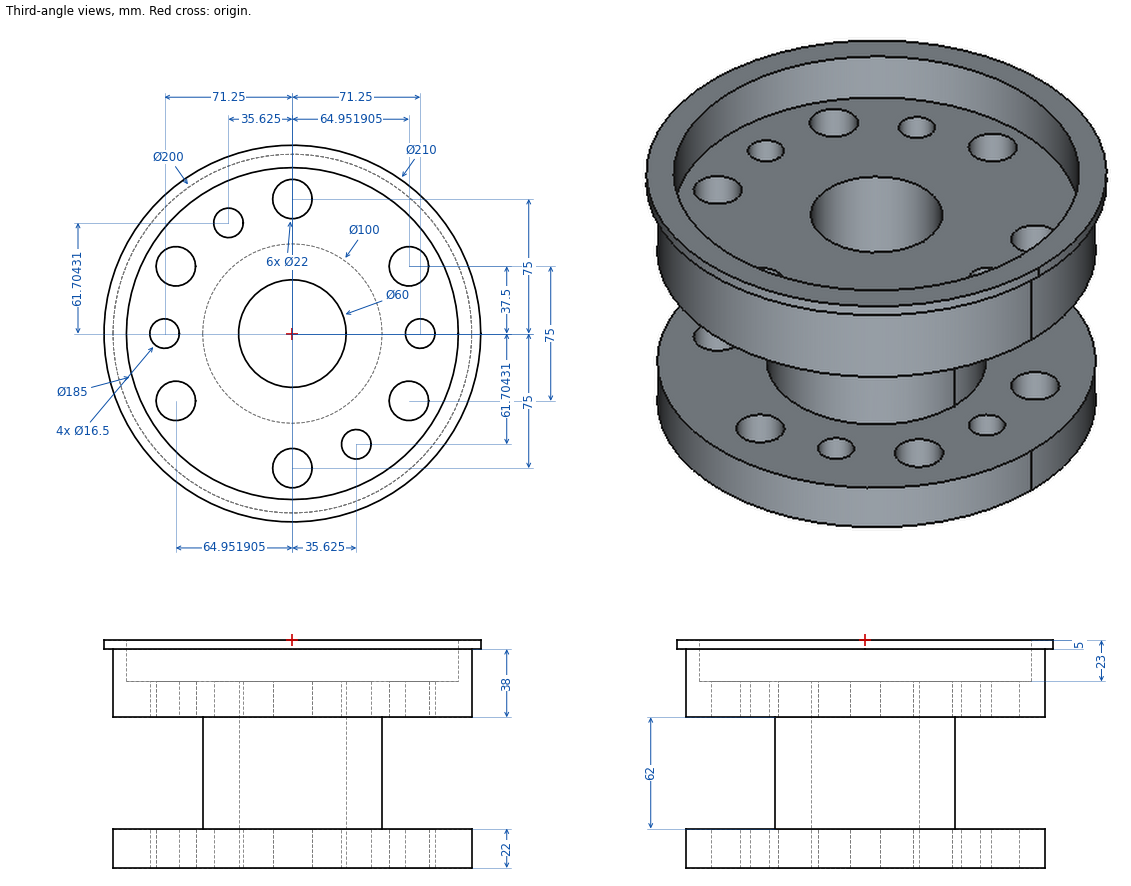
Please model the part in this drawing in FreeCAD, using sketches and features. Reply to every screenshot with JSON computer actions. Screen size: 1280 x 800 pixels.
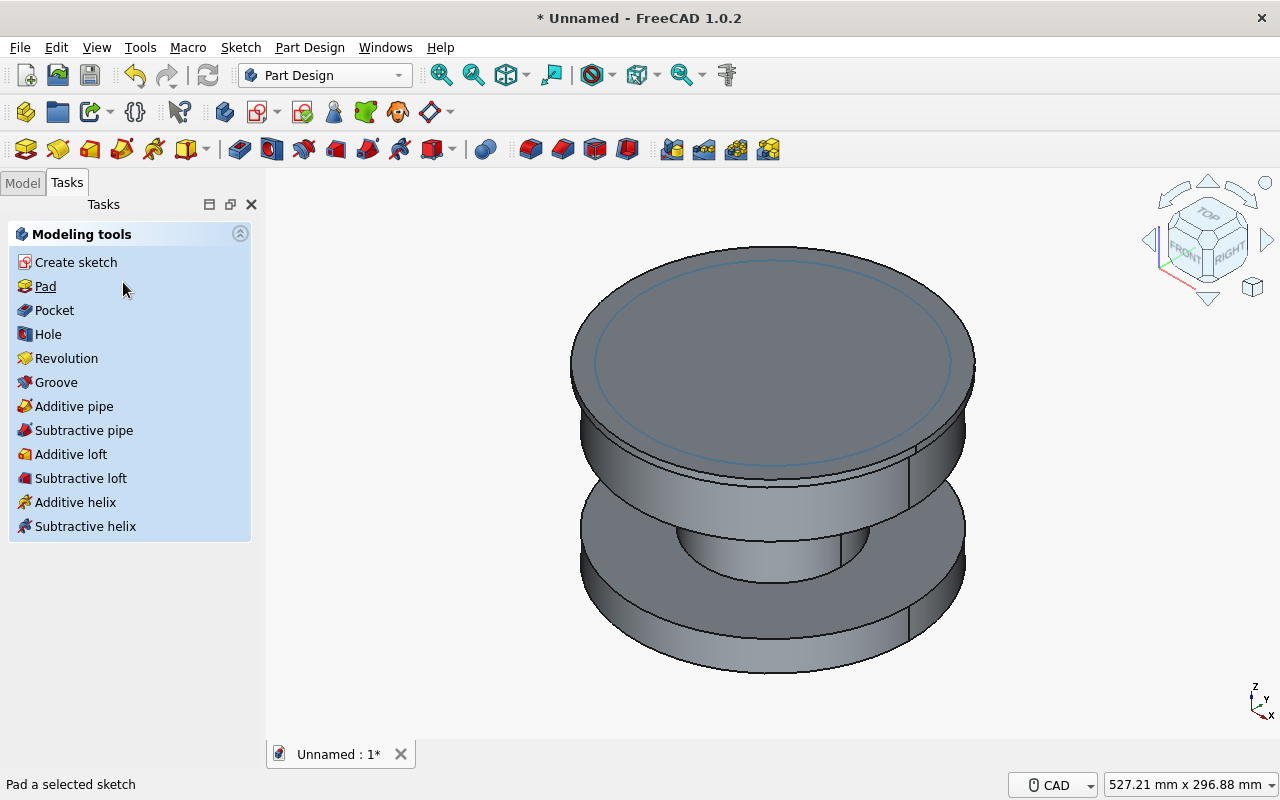
{"action": "left_click", "coordinate": [240, 150]}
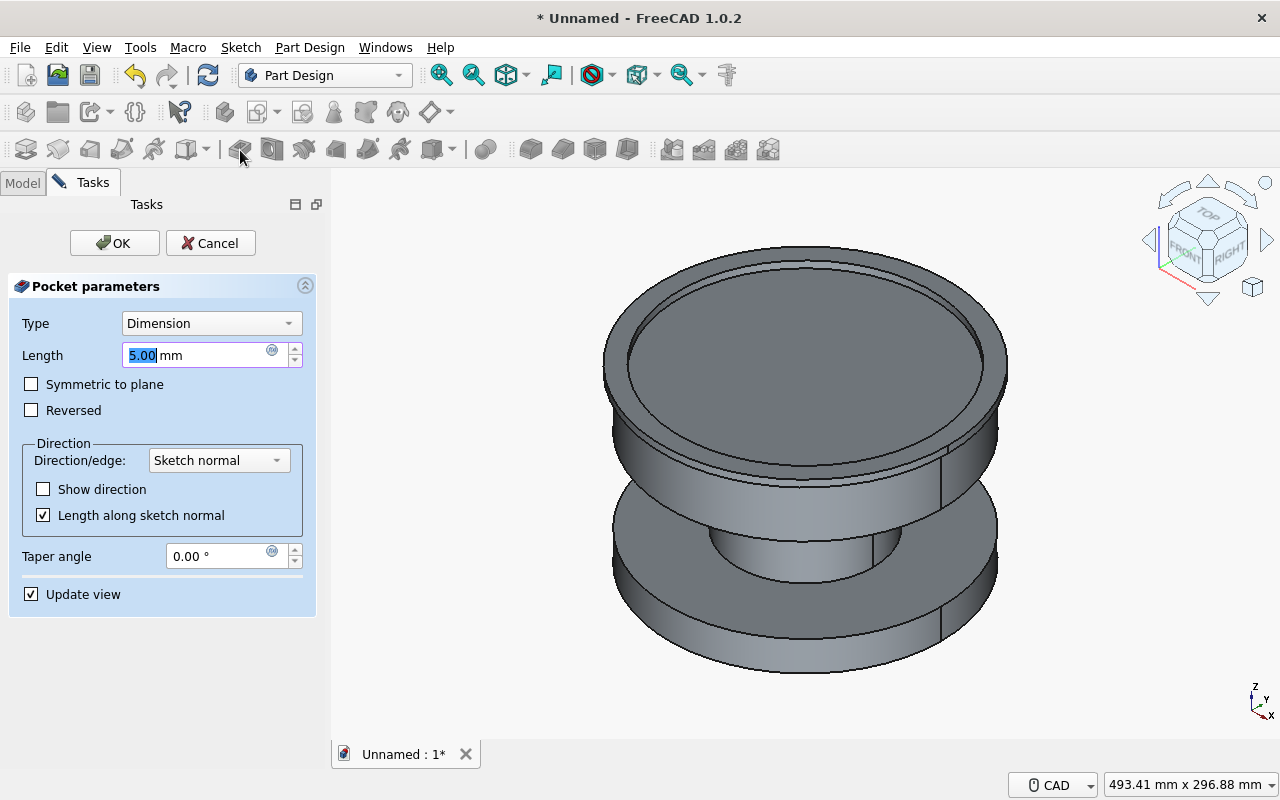
{"action": "type", "text": "23"}
{"action": "key", "text": "Tab"}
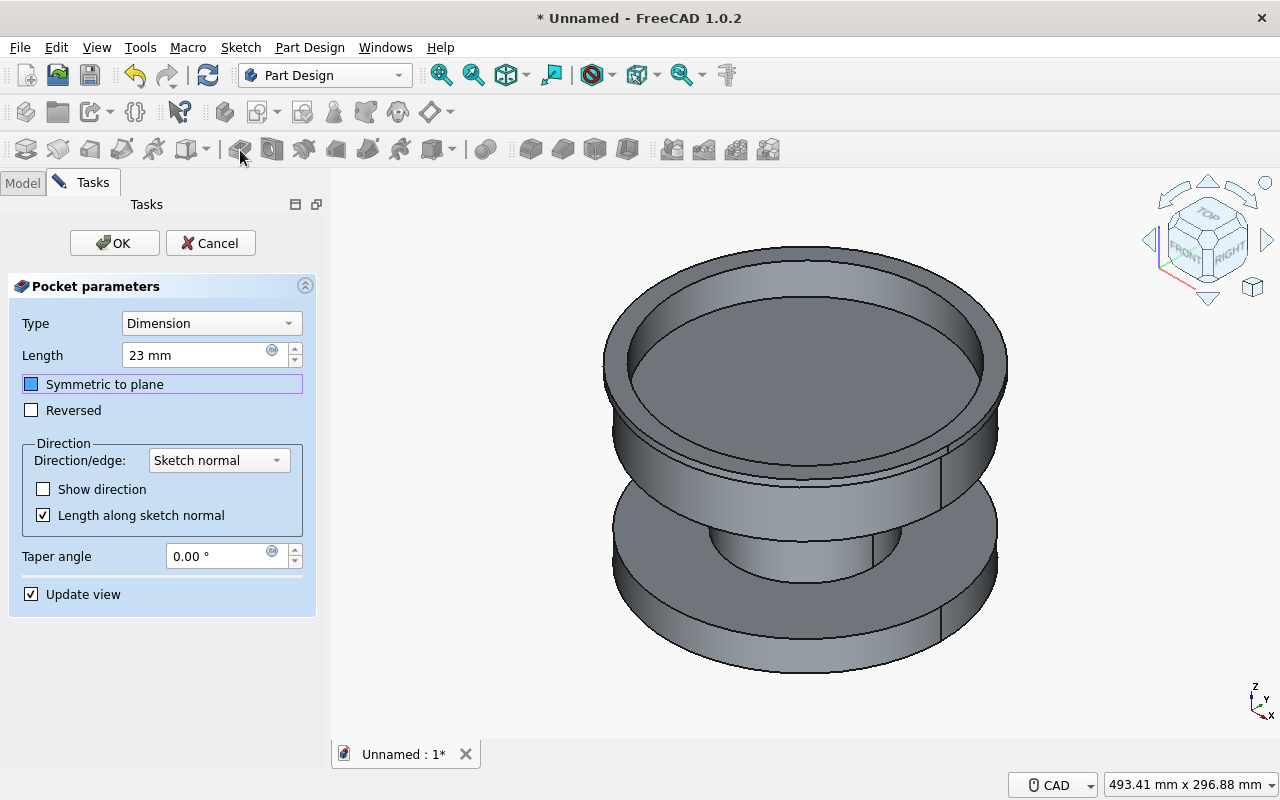
{"action": "left_click", "coordinate": [115, 243]}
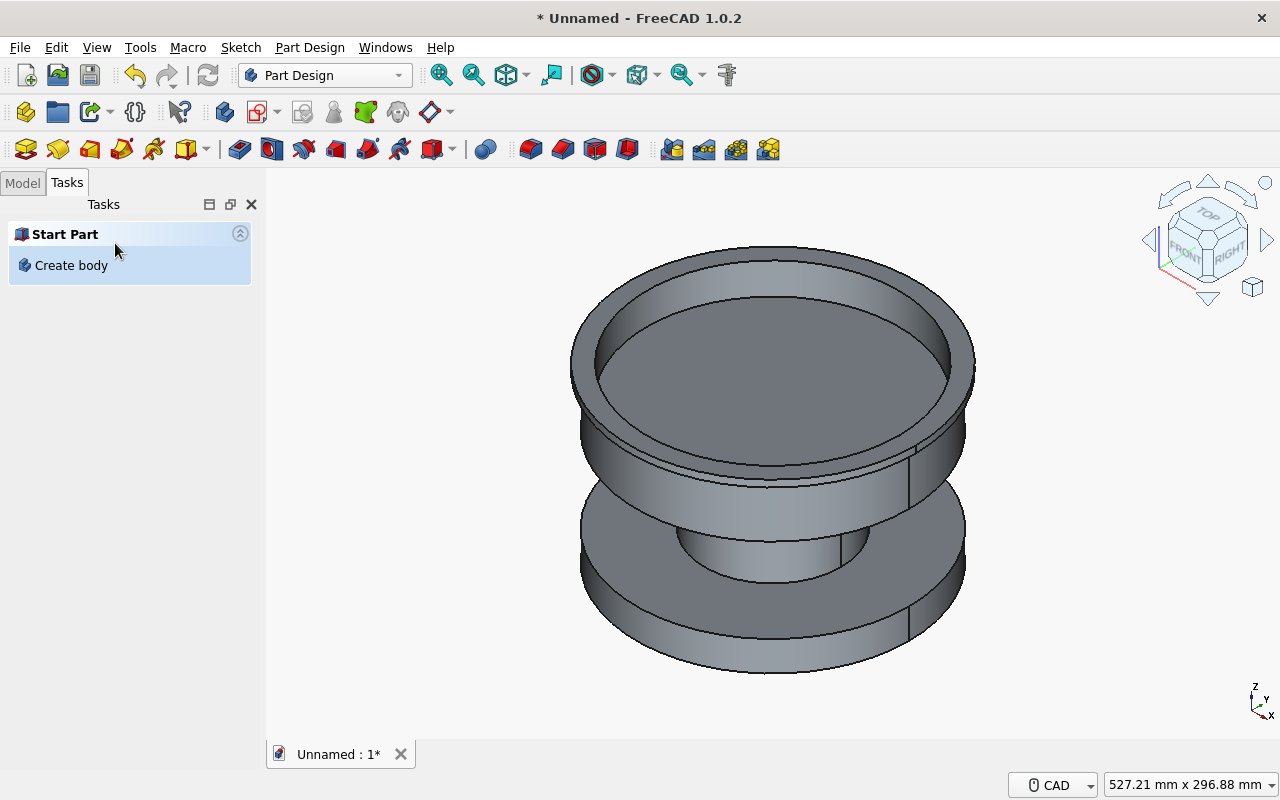
{"action": "left_click", "coordinate": [773, 398]}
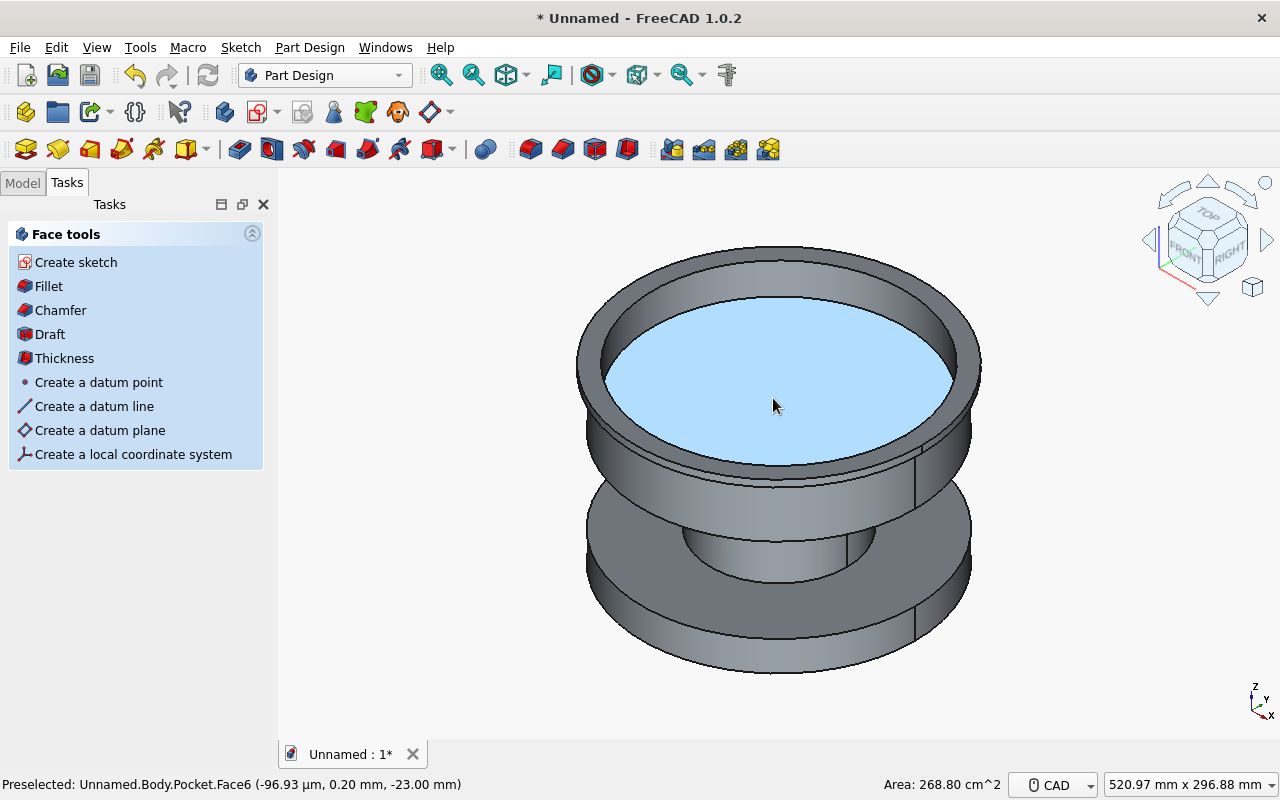
{"action": "left_click", "coordinate": [258, 112]}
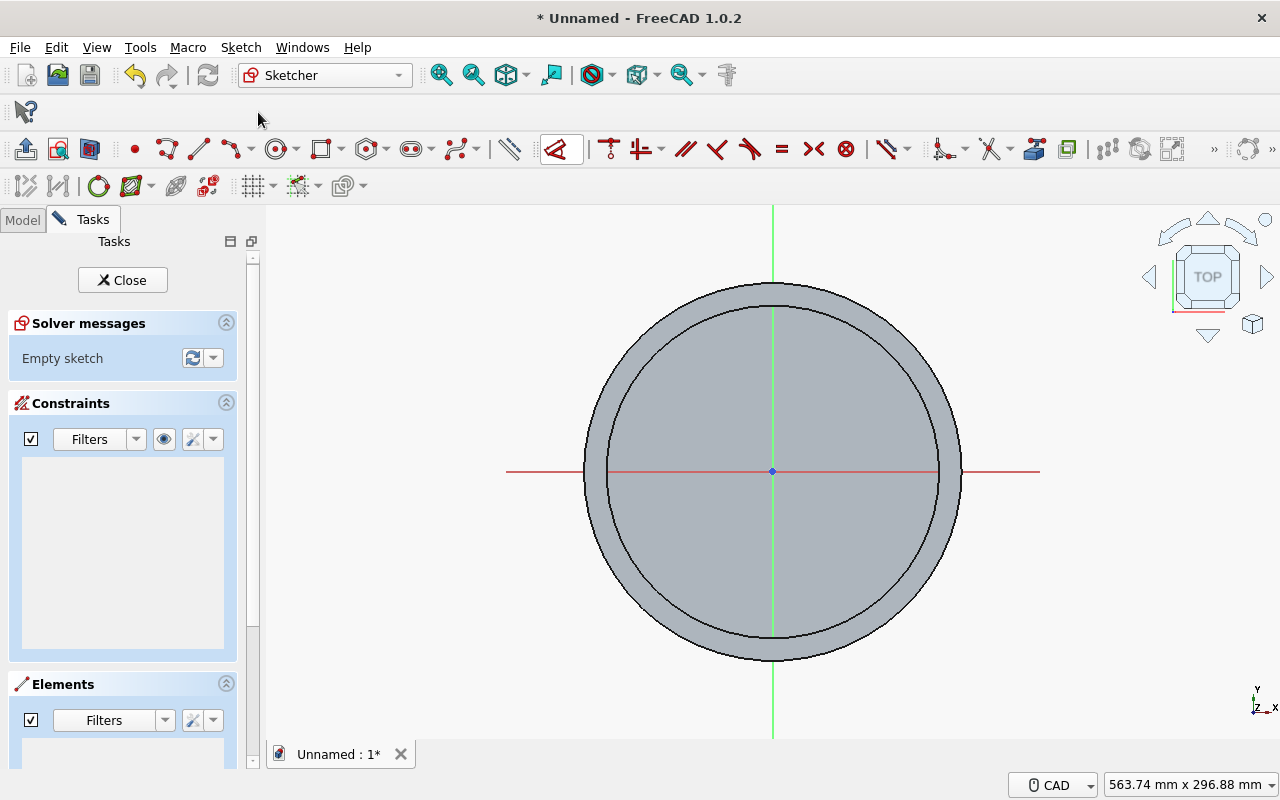
{"action": "left_click", "coordinate": [90, 150]}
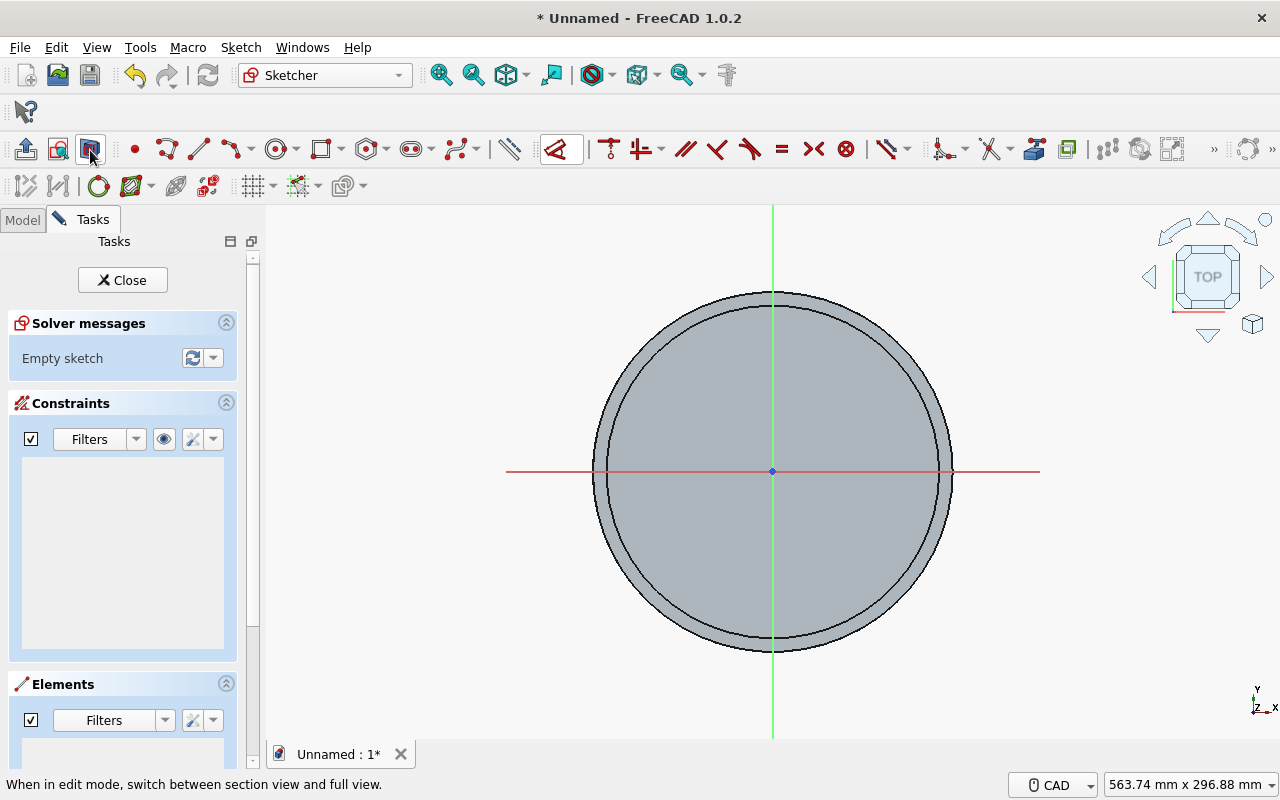
{"action": "scroll", "coordinate": [802, 472], "scroll_direction": "up", "scroll_amount": 6}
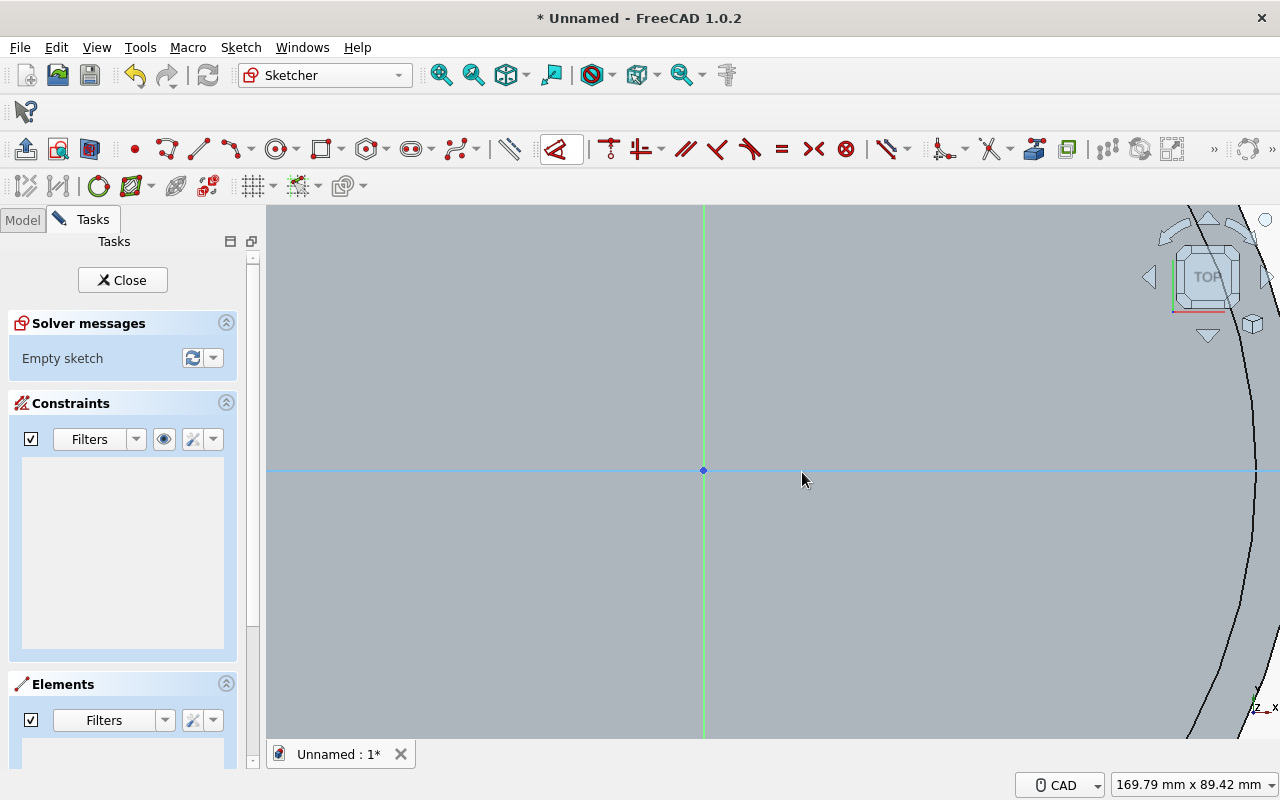
{"action": "left_click", "coordinate": [276, 150]}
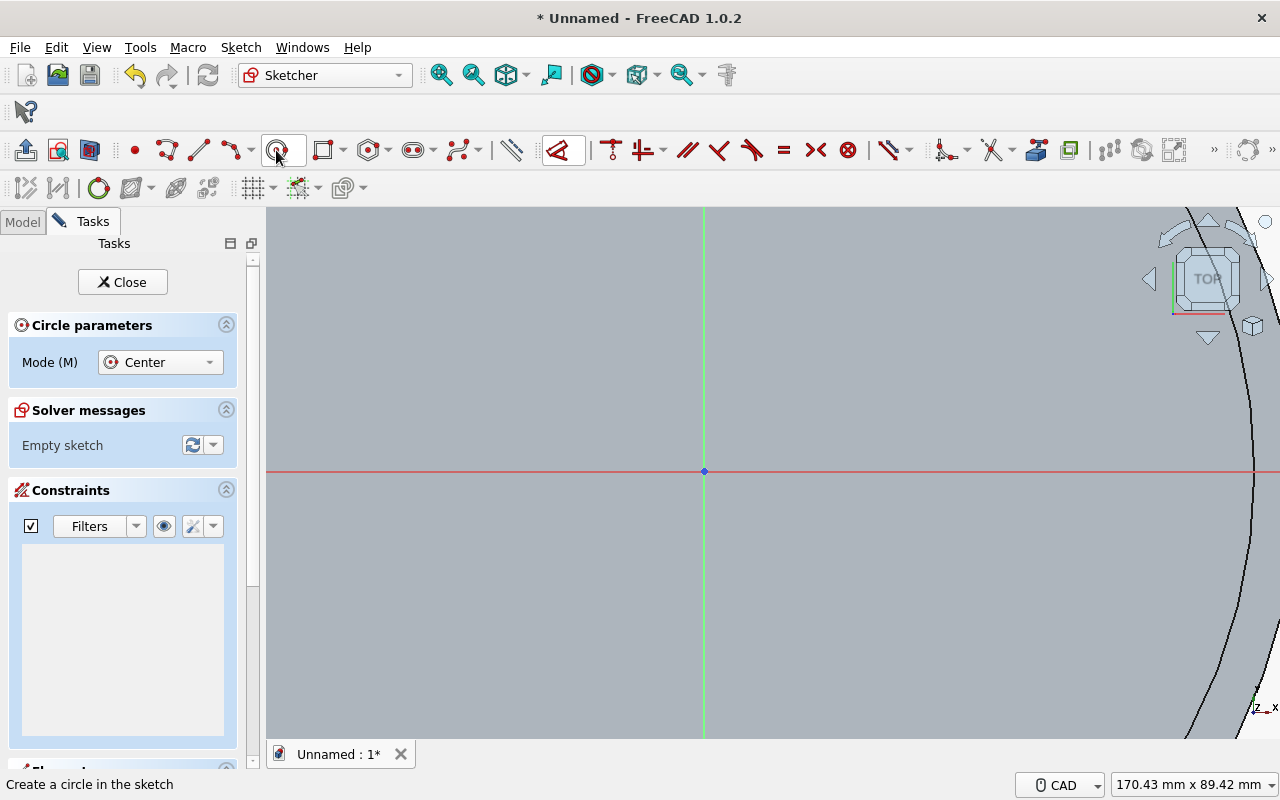
{"action": "left_click", "coordinate": [704, 472]}
{"action": "mouse_move", "coordinate": [830, 346]}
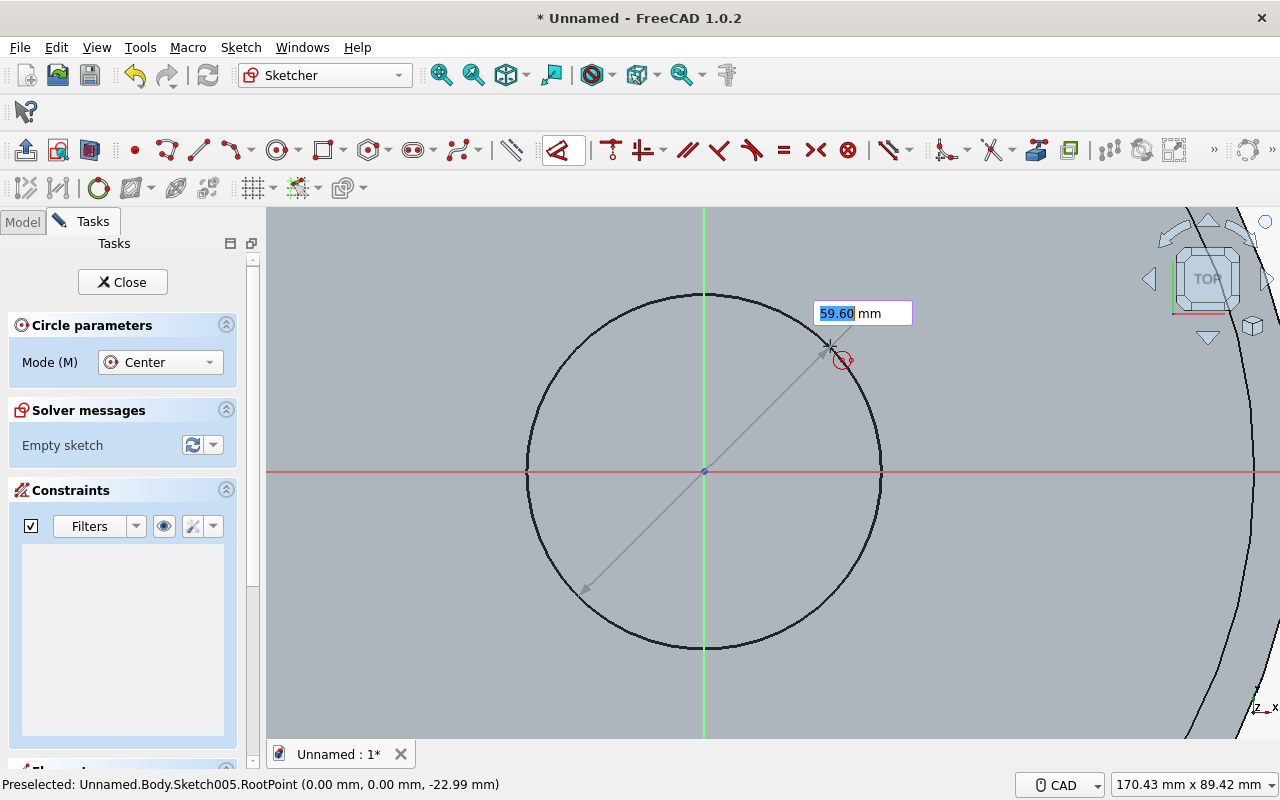
{"action": "type", "text": "60"}
{"action": "key", "text": "Return"}
{"action": "key", "text": "Escape"}